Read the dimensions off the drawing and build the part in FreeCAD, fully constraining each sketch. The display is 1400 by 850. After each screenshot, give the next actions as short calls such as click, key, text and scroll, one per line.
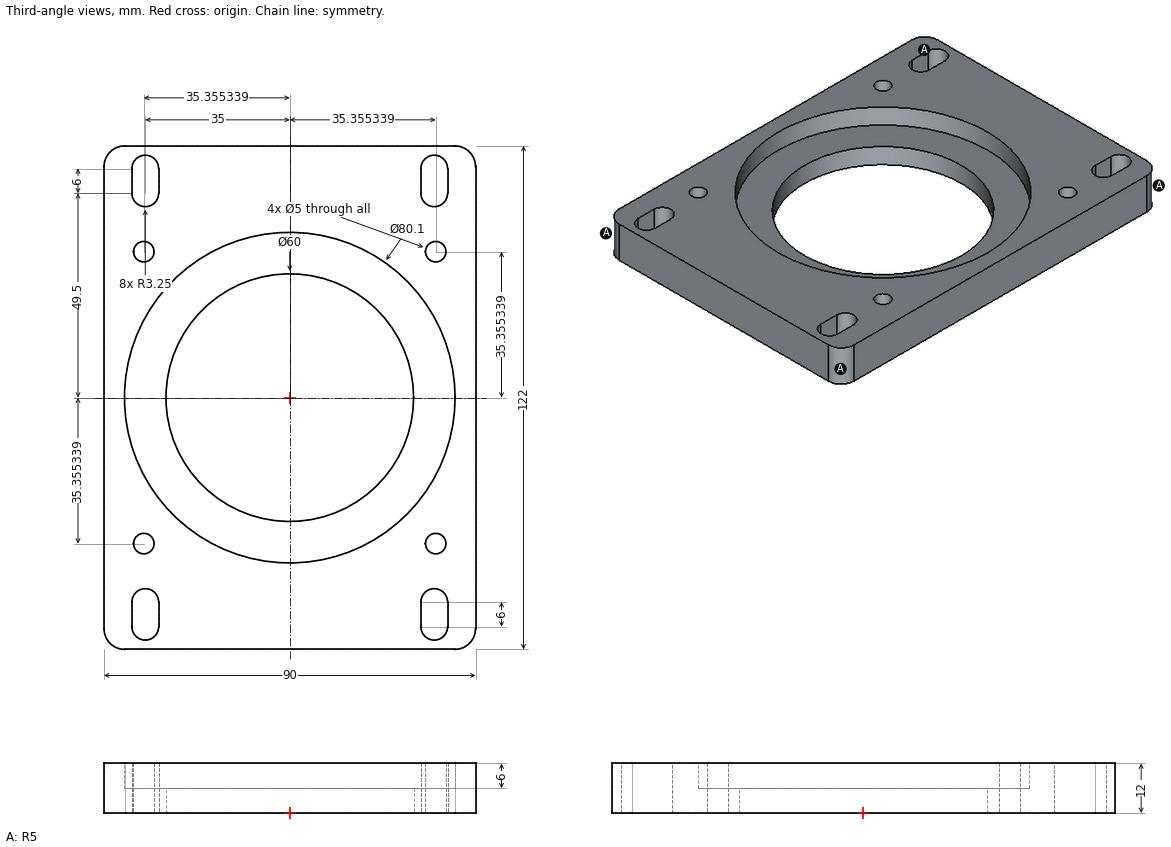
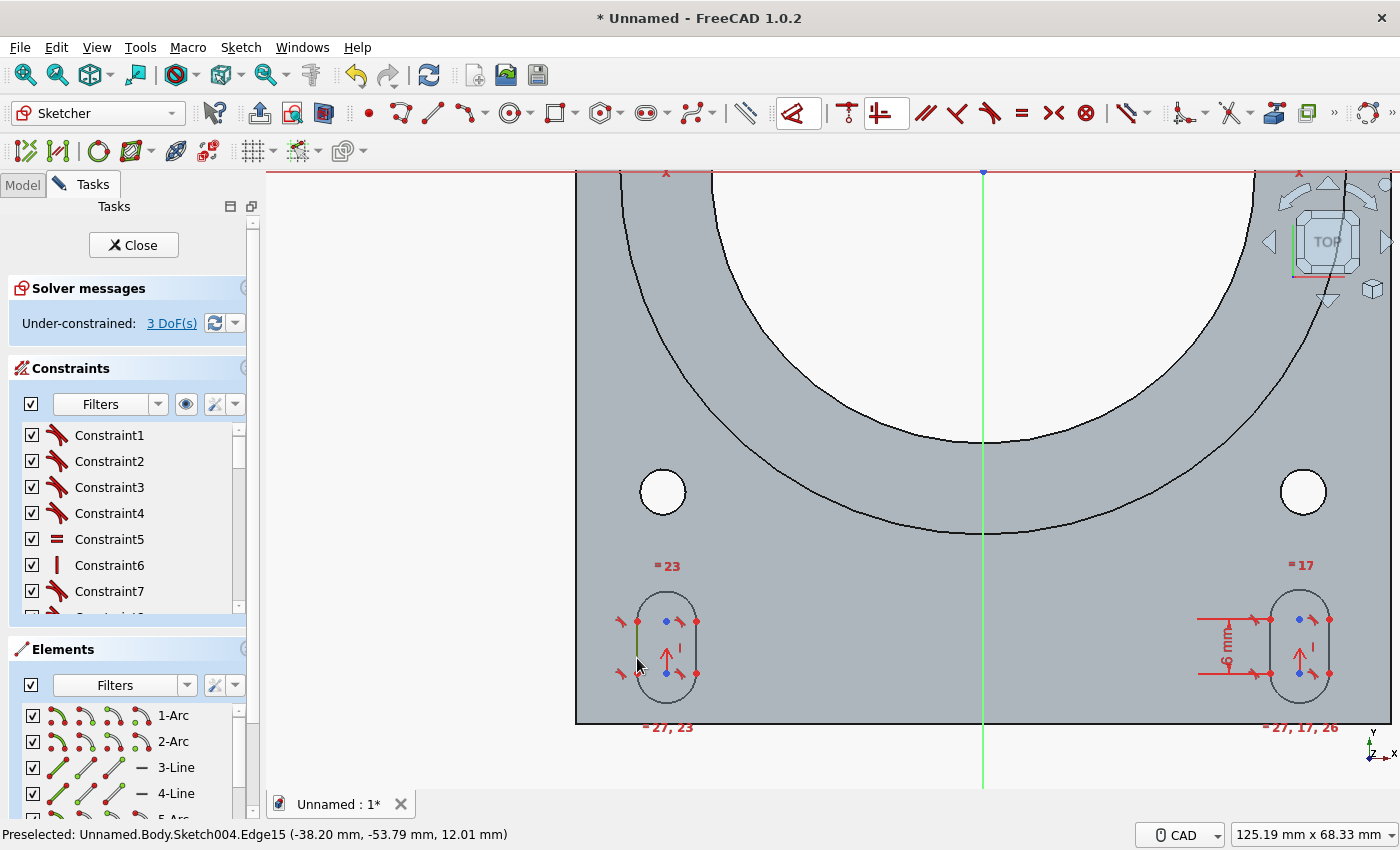
key(i)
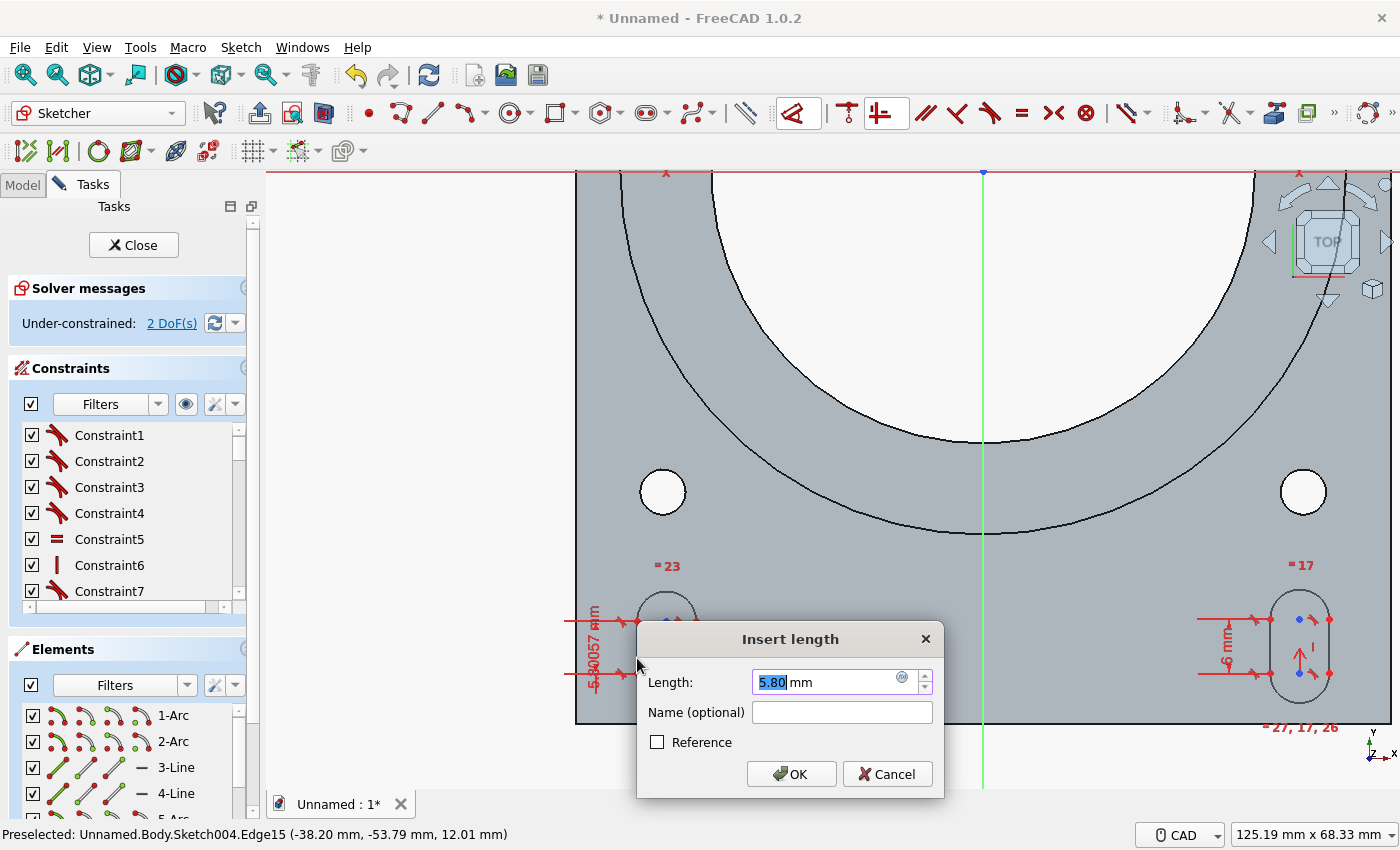
text(6)
key(Return)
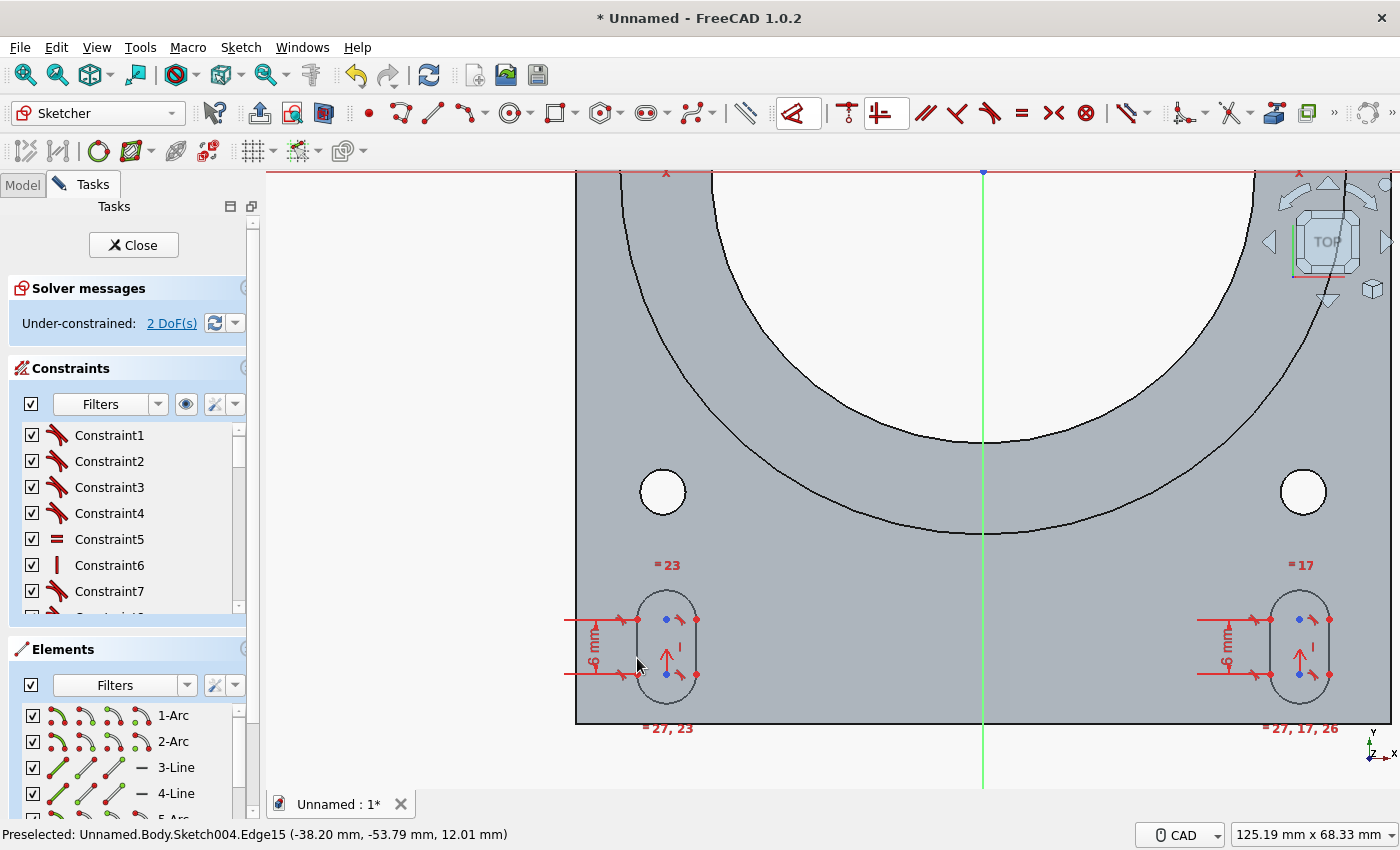
scroll(637, 659, down, 5)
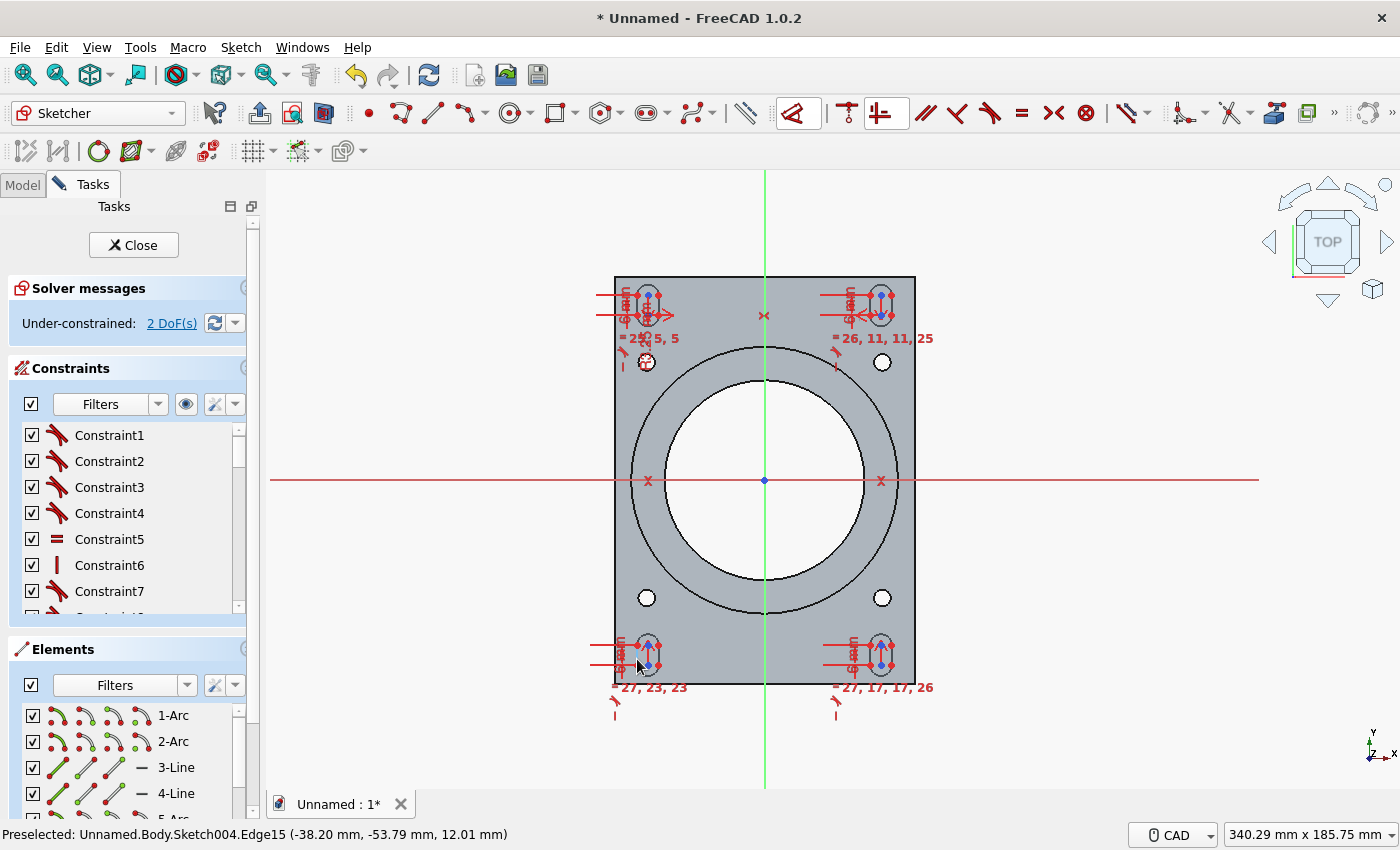
click(648, 315)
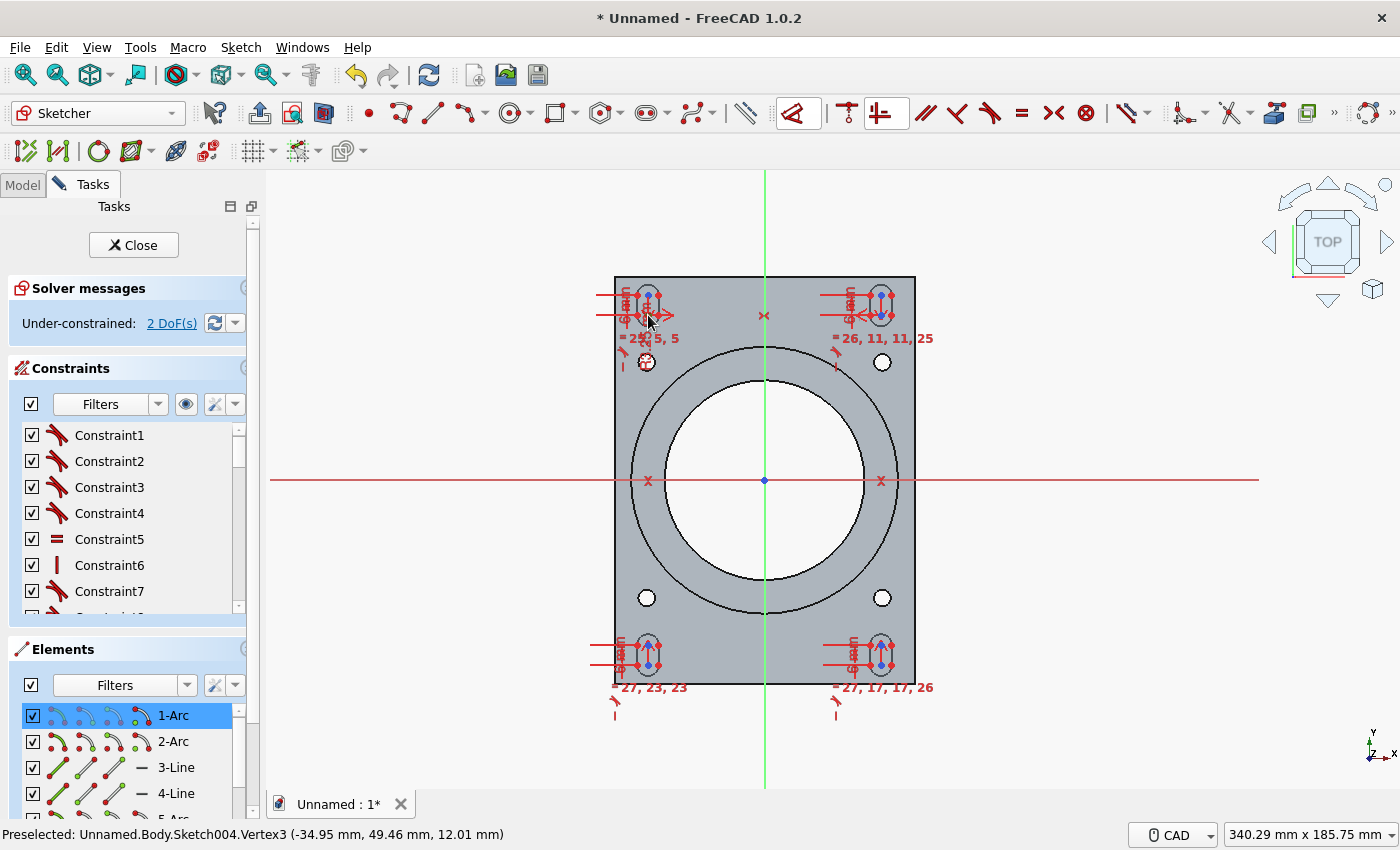
click(816, 114)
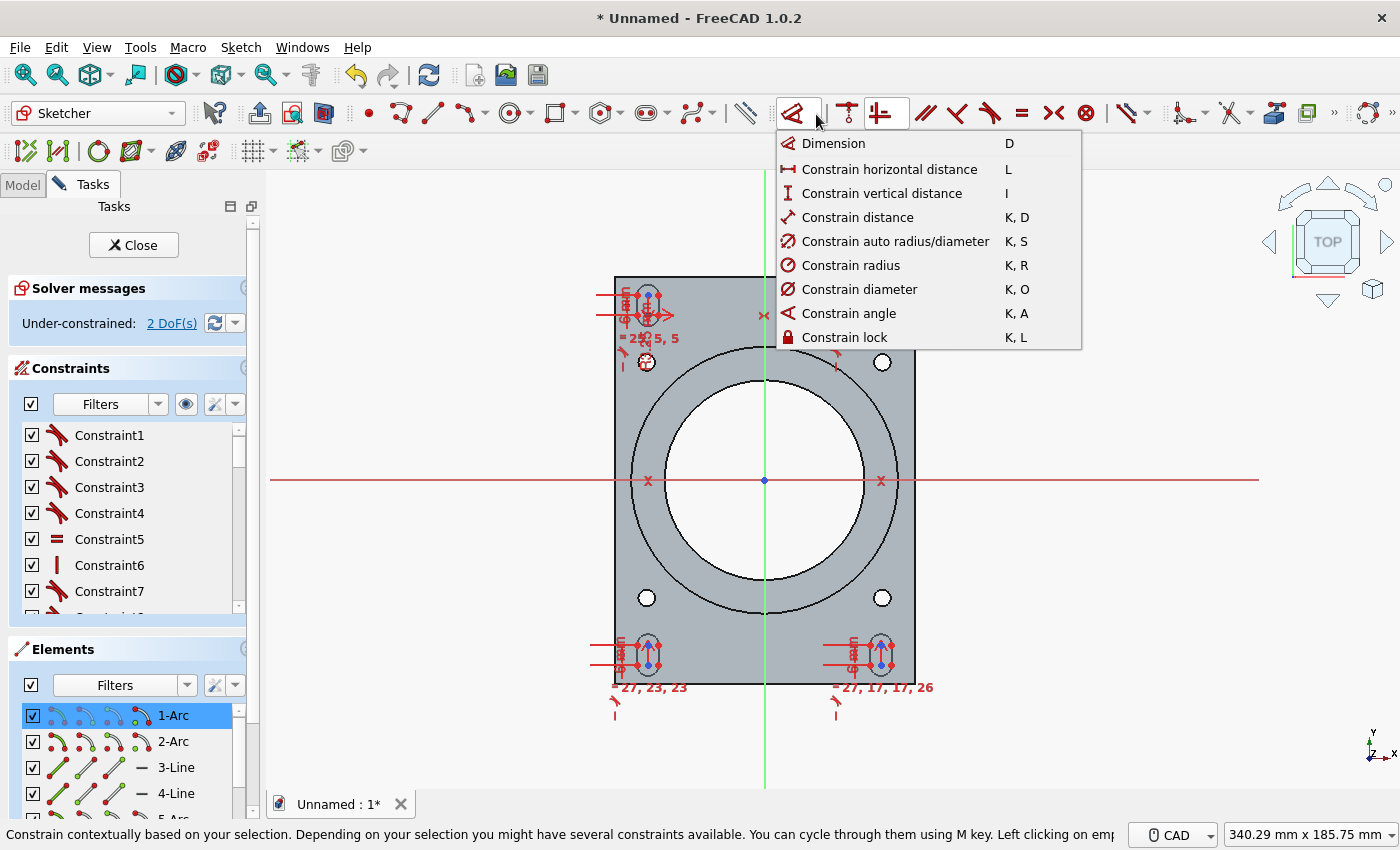
click(929, 169)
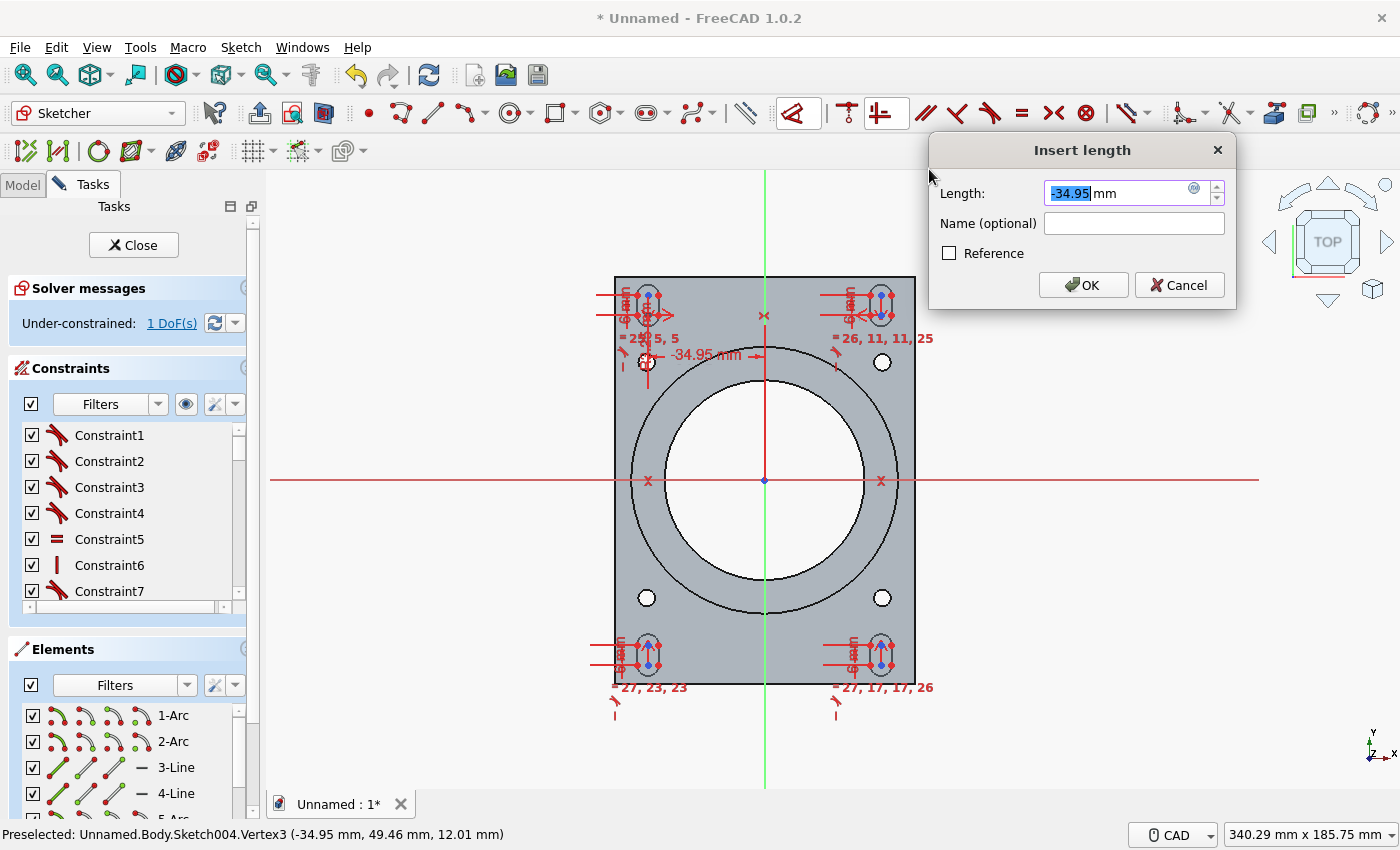
text(-35)
key(Return)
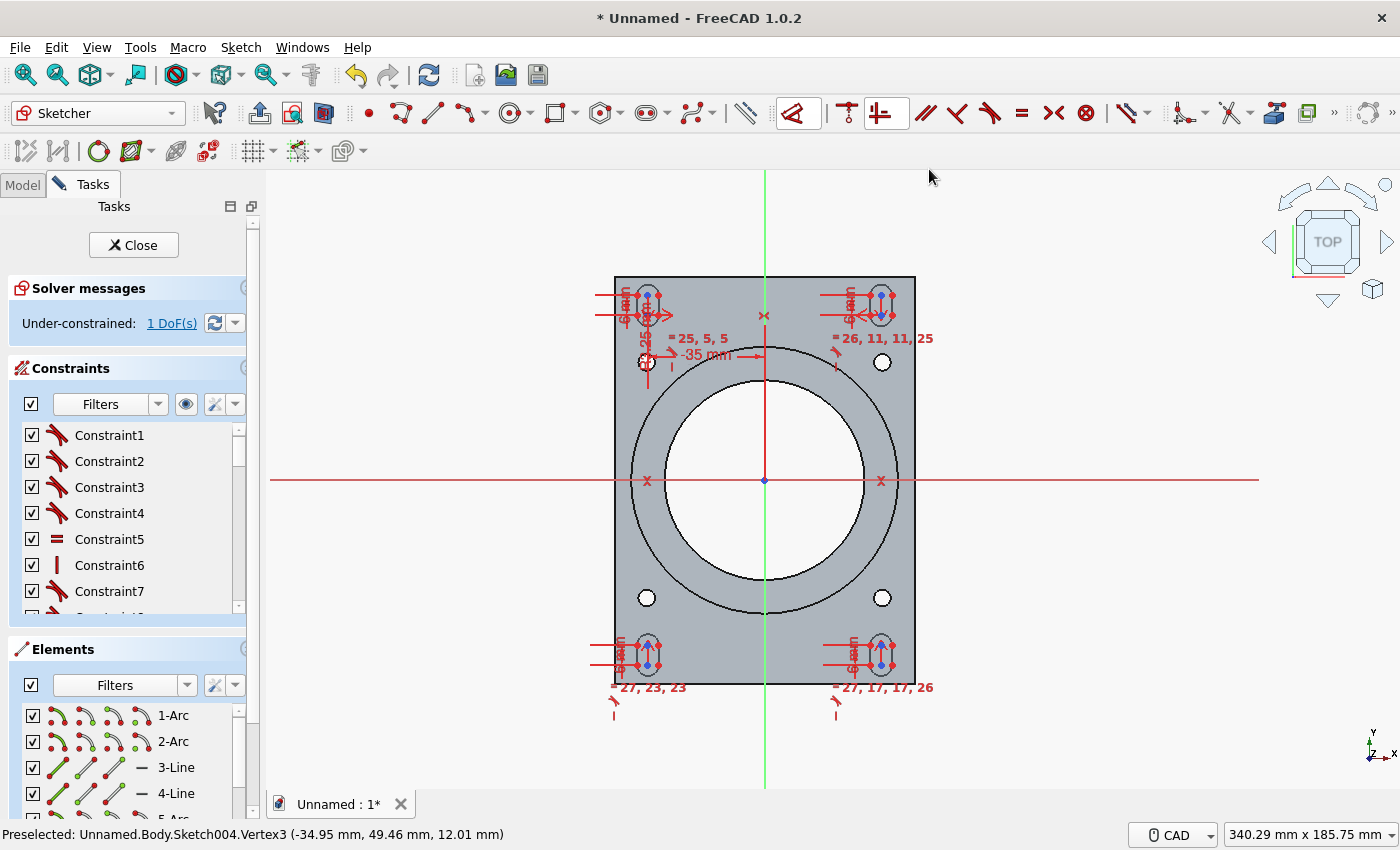
click(637, 315)